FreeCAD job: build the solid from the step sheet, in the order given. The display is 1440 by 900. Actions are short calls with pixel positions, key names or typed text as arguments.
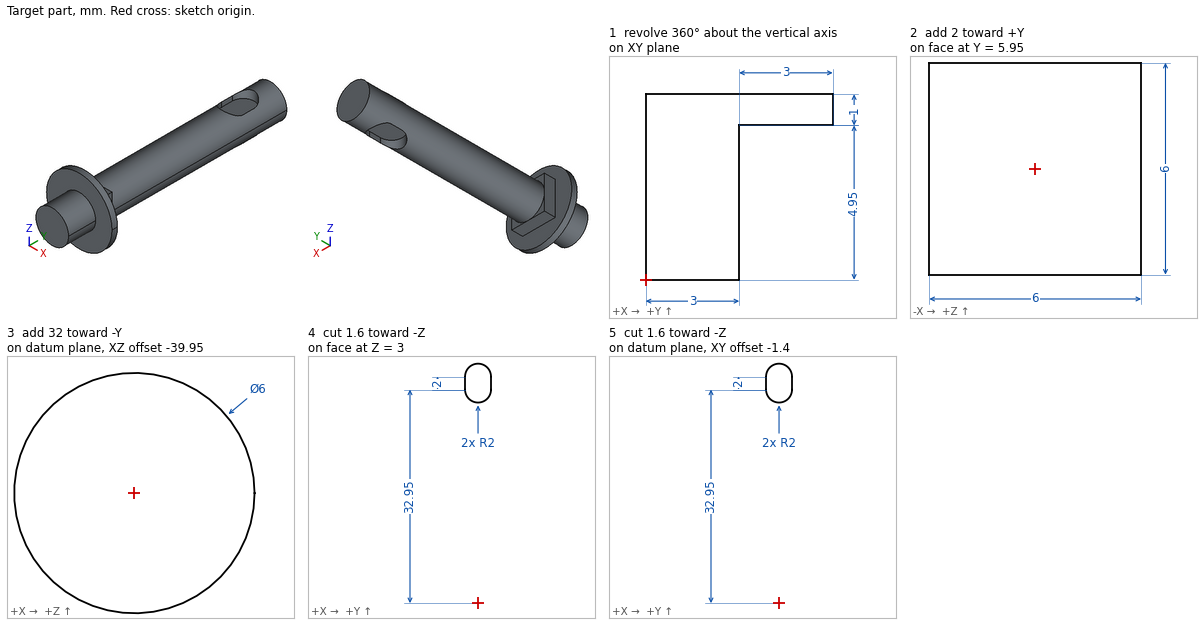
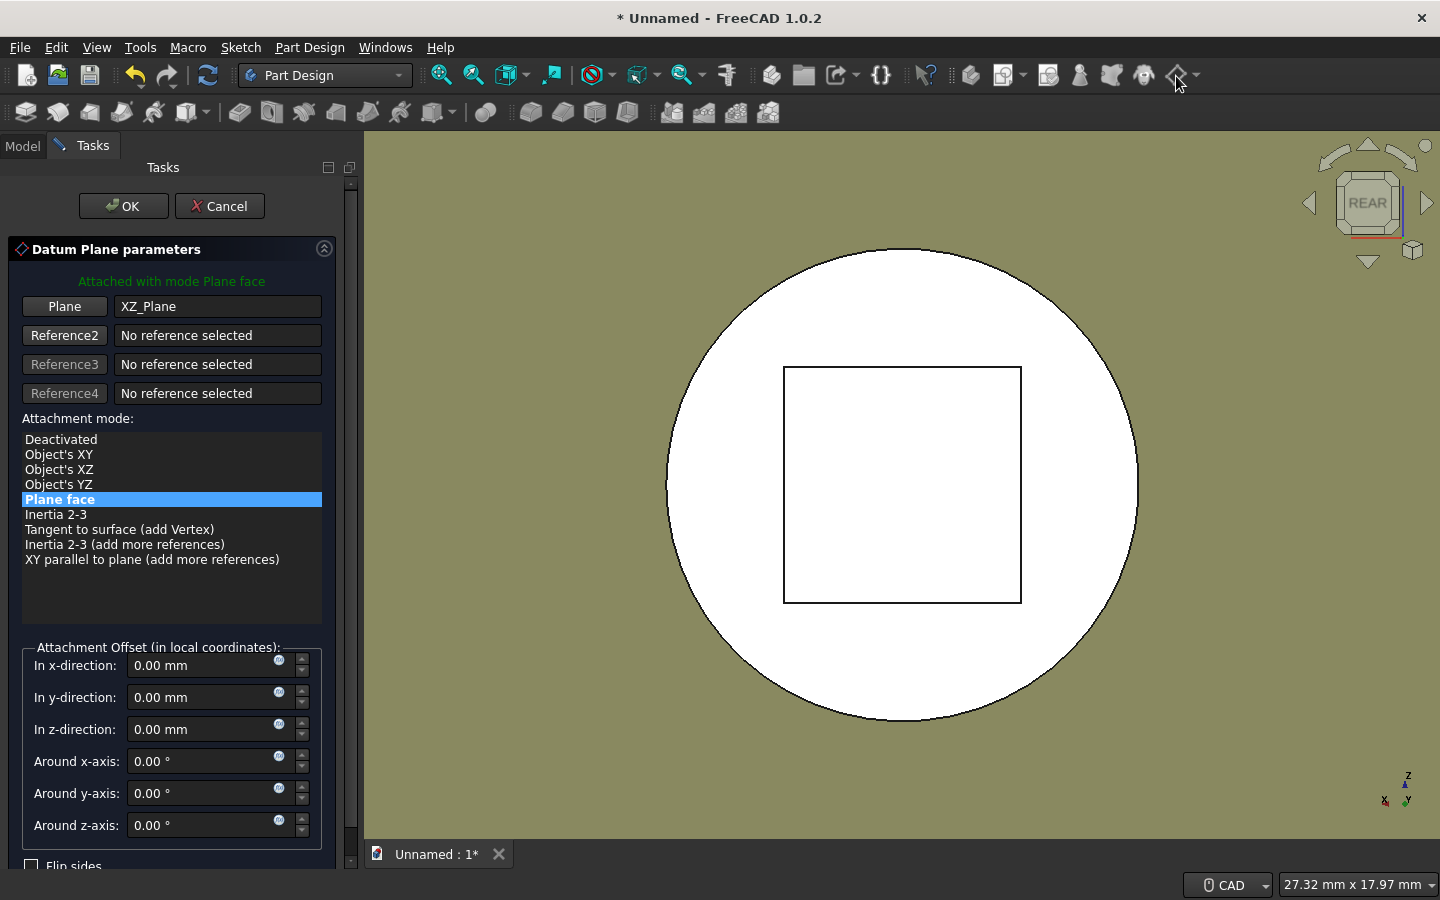
triple_click(210, 729)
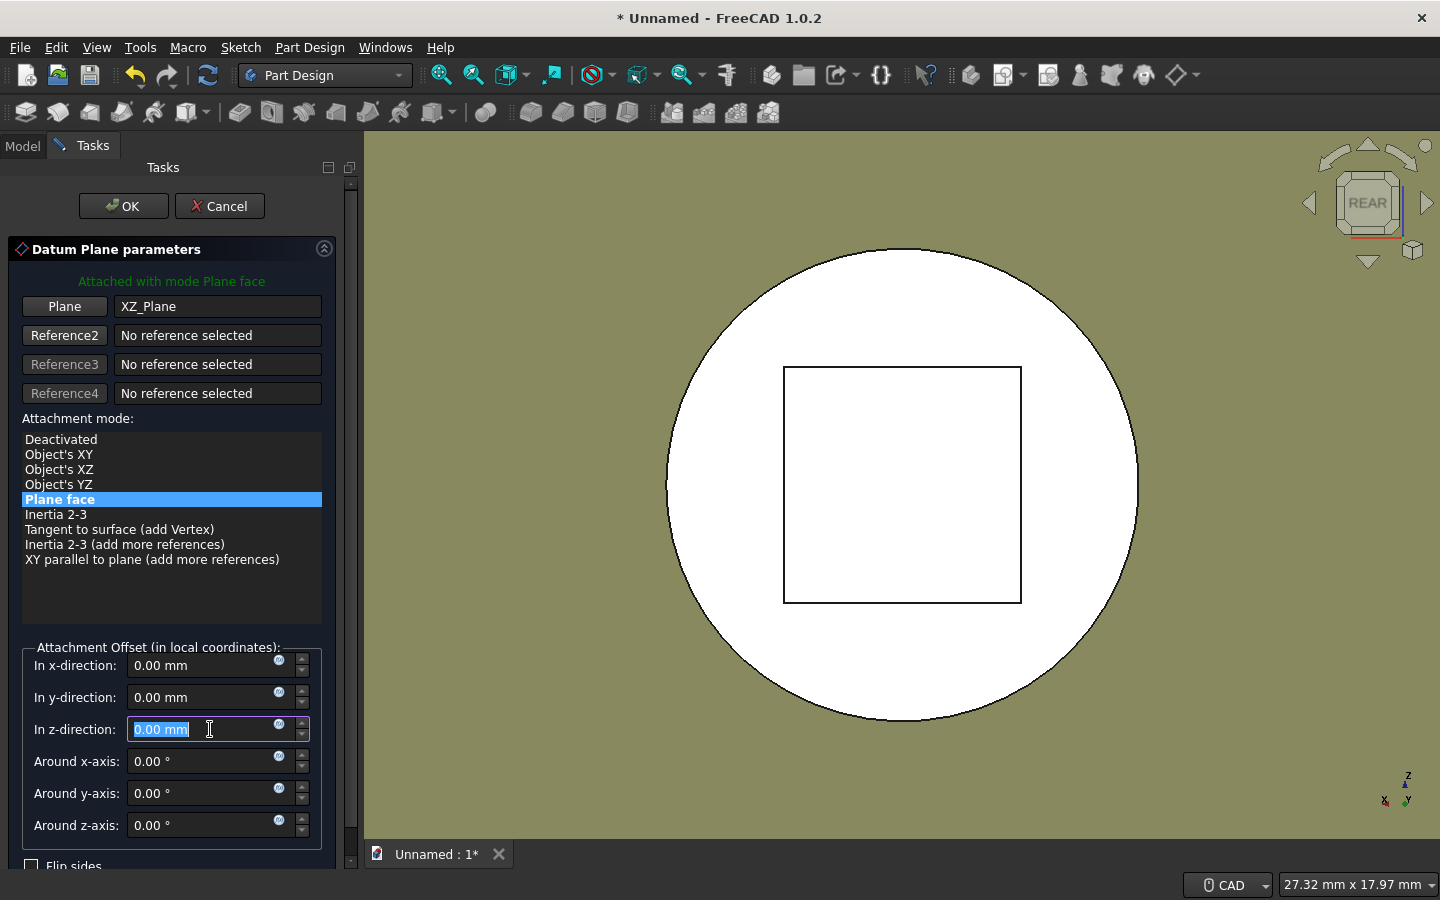
text(-39.95)
key(Tab)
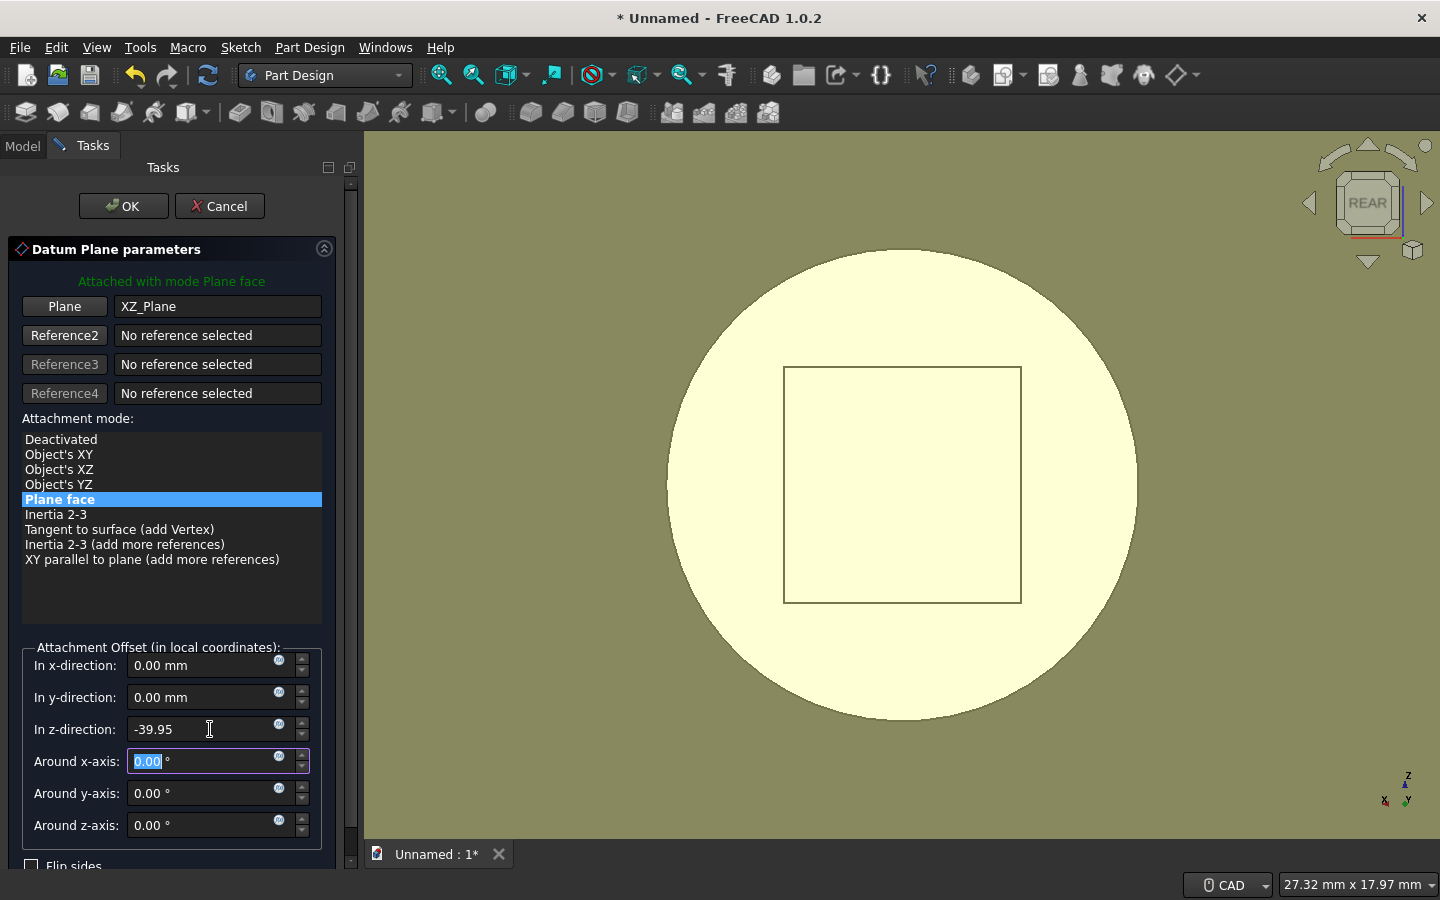
click(124, 206)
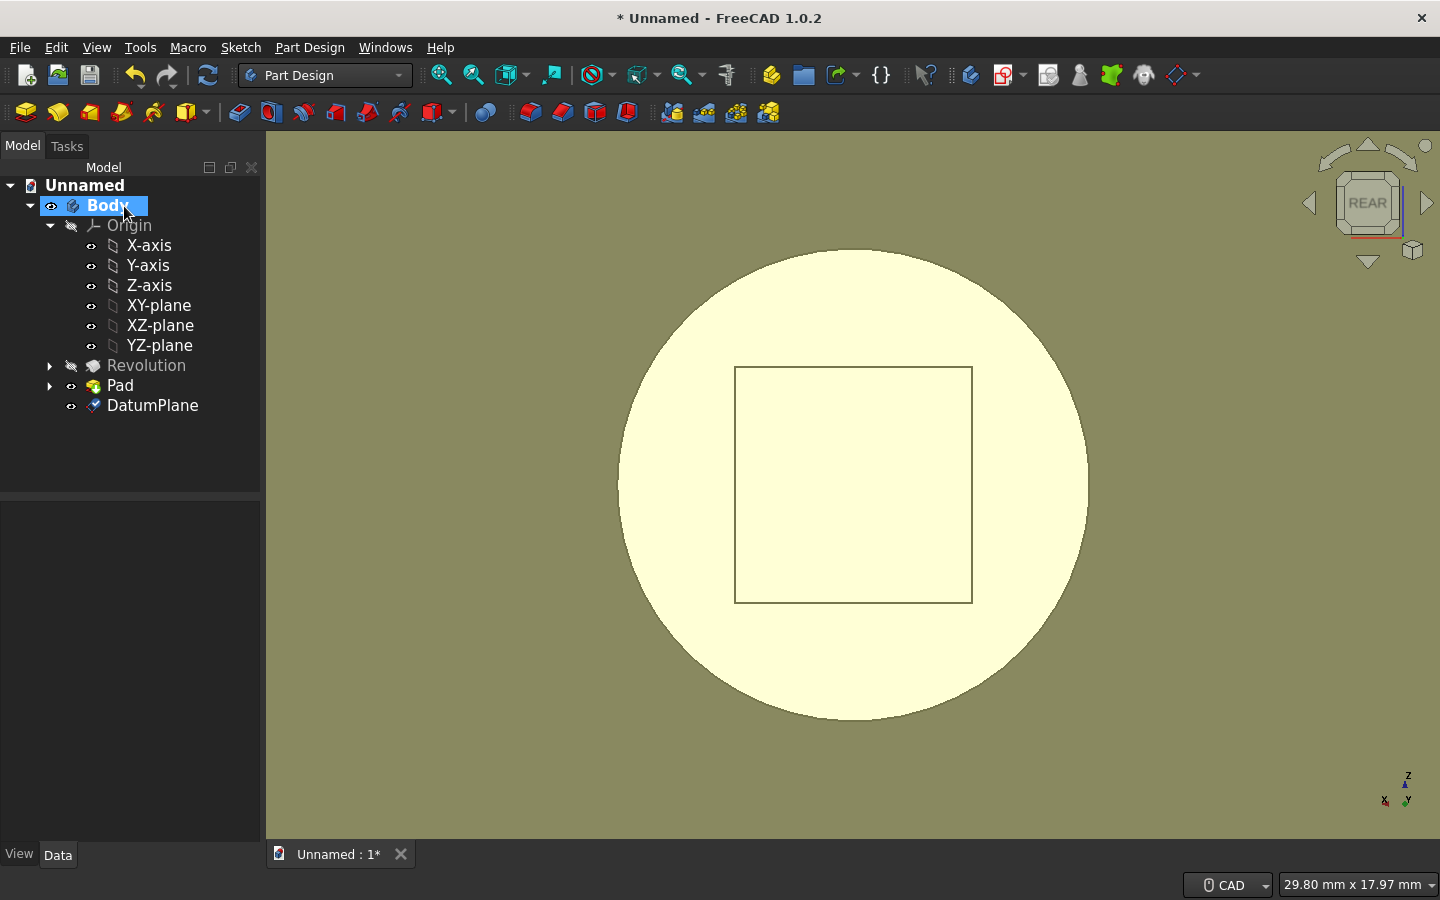
click(116, 406)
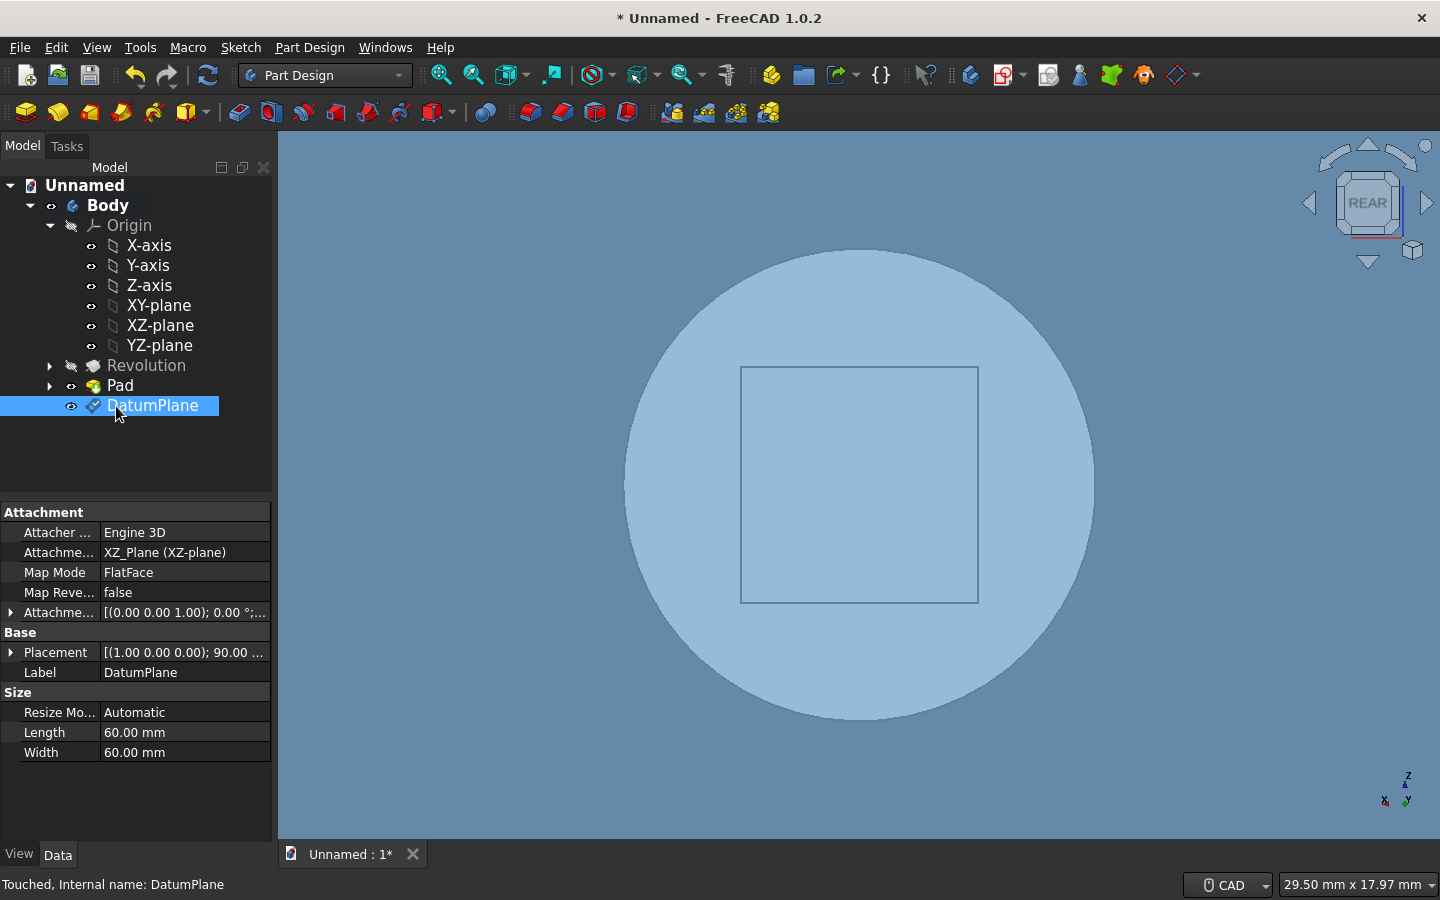
click(1004, 76)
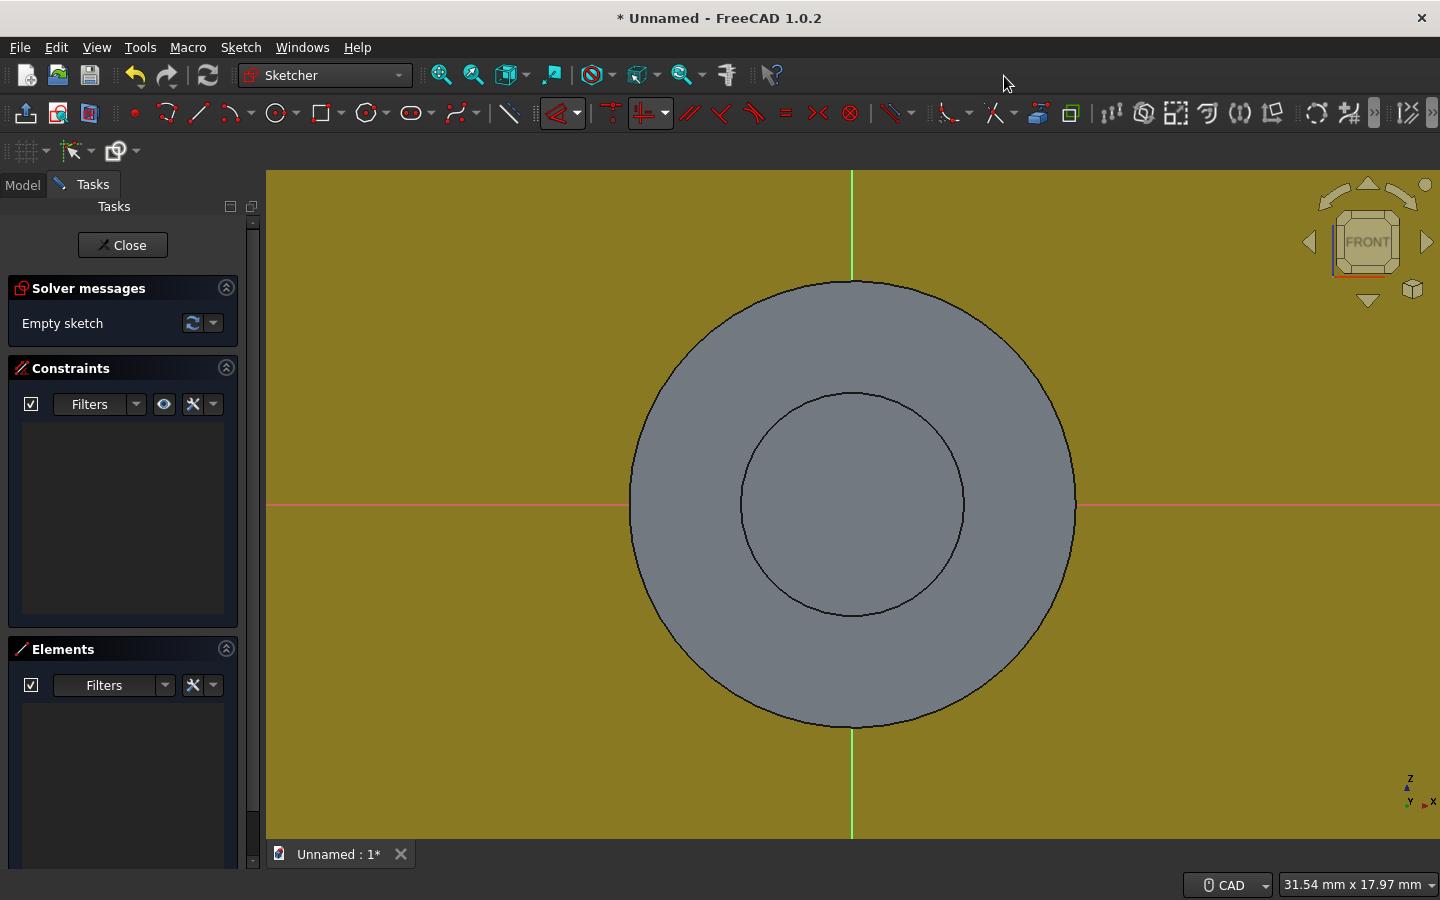
key(q)
key(s)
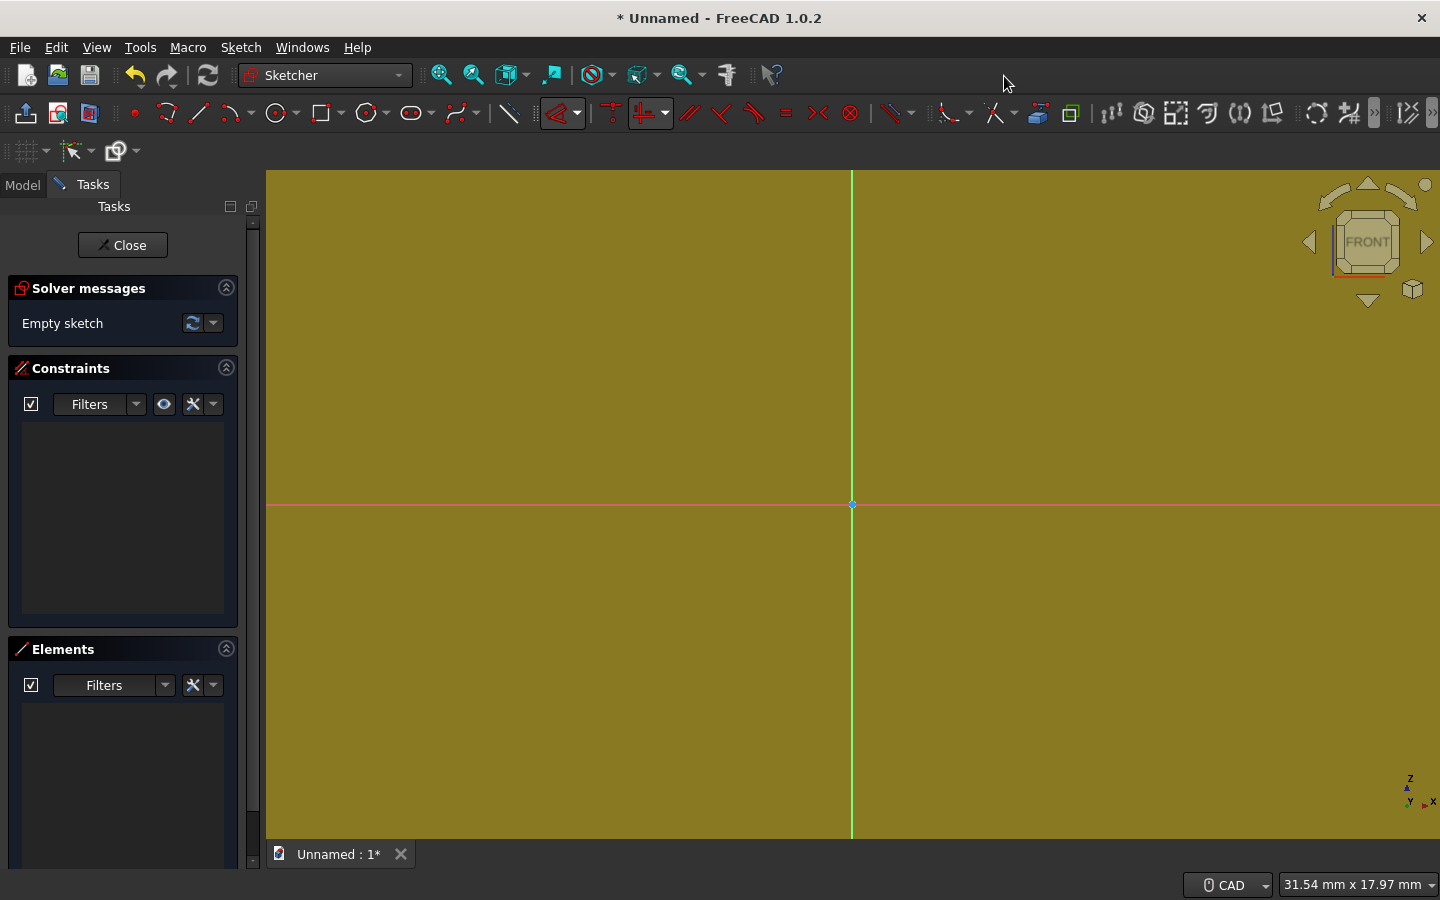
scroll(935, 505, up, 3)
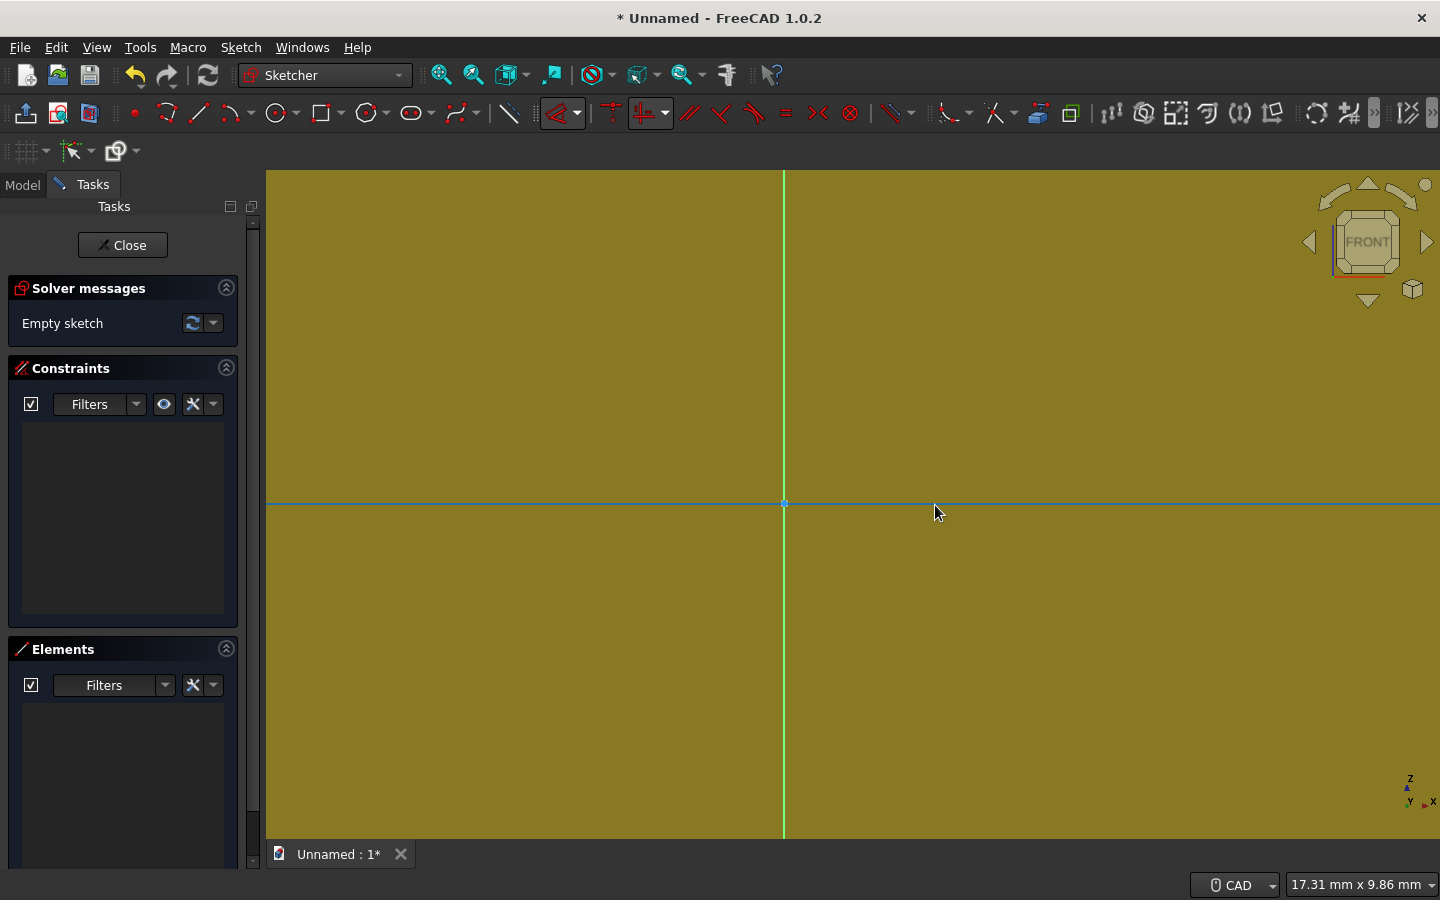
click(276, 114)